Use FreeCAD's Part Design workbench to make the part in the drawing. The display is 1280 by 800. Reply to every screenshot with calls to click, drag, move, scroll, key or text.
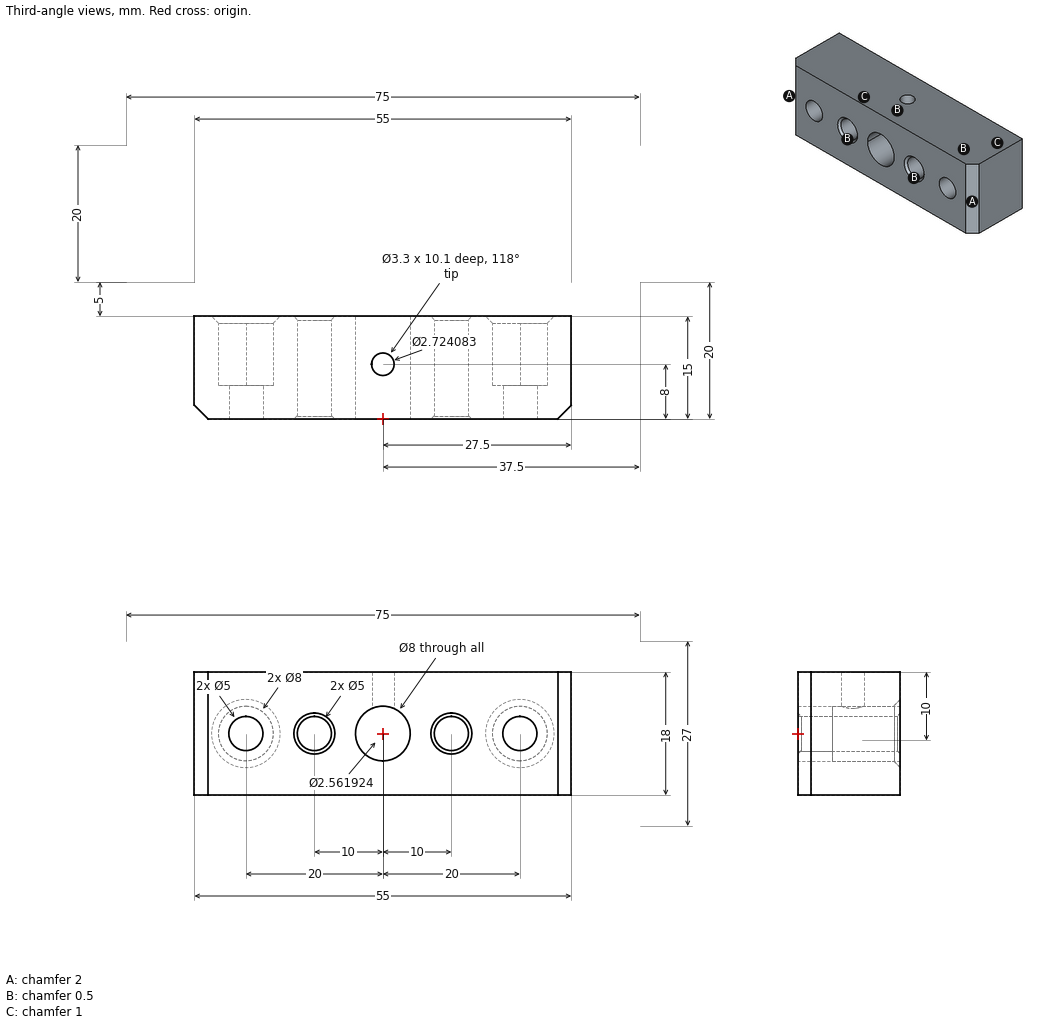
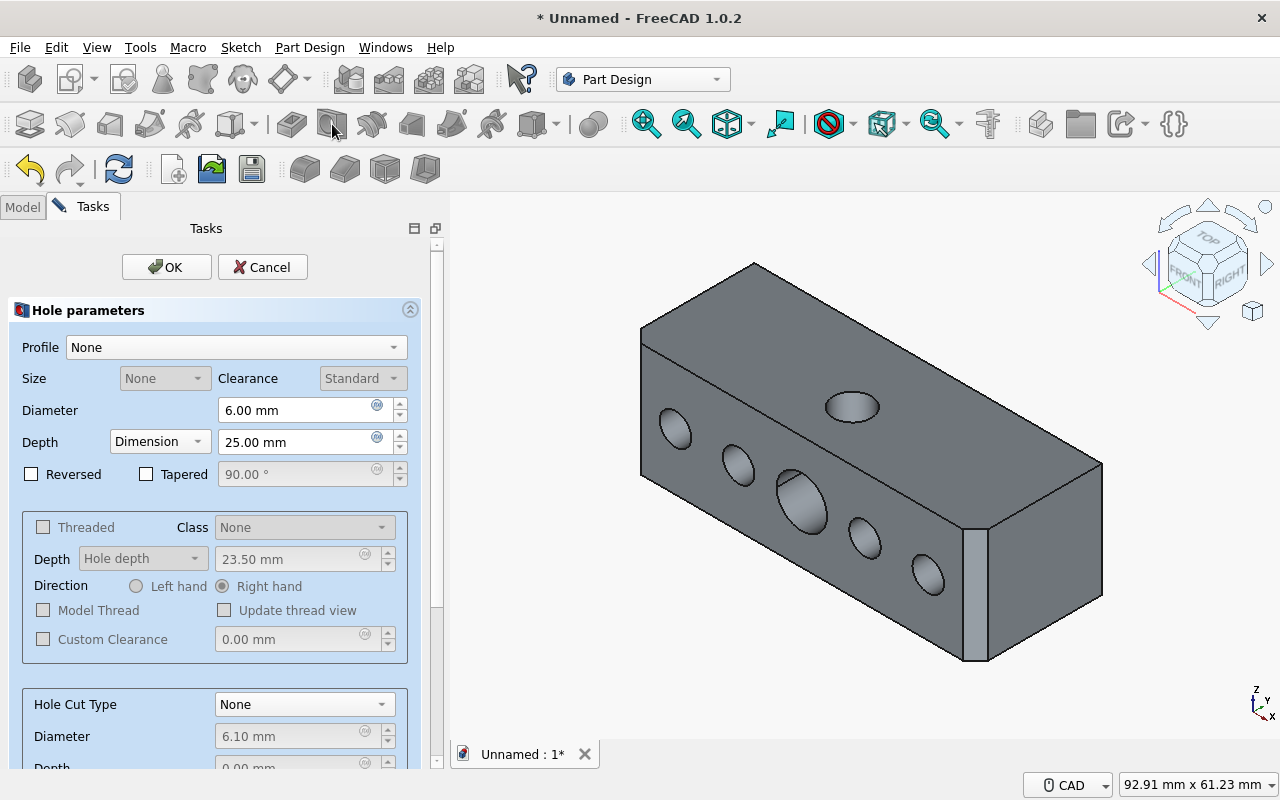
triple_click(305, 410)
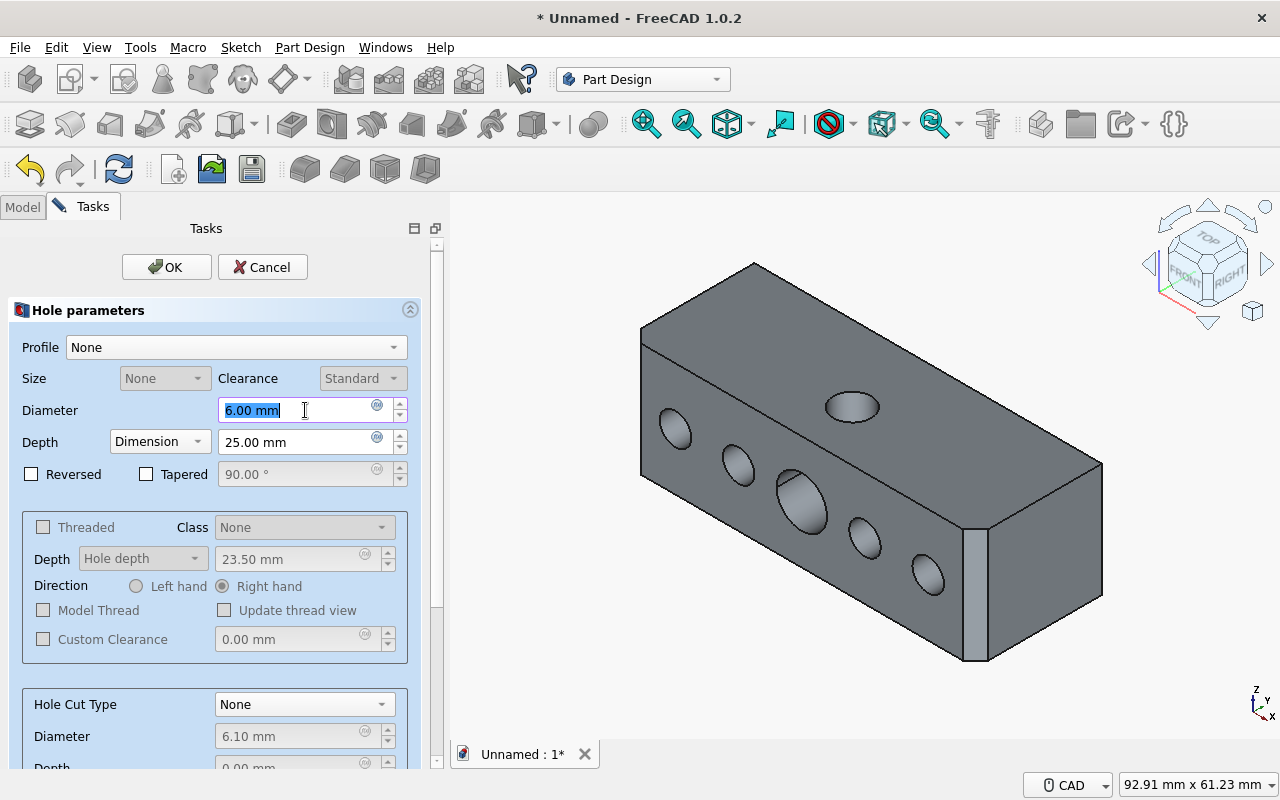
text(3.3)
key(Tab)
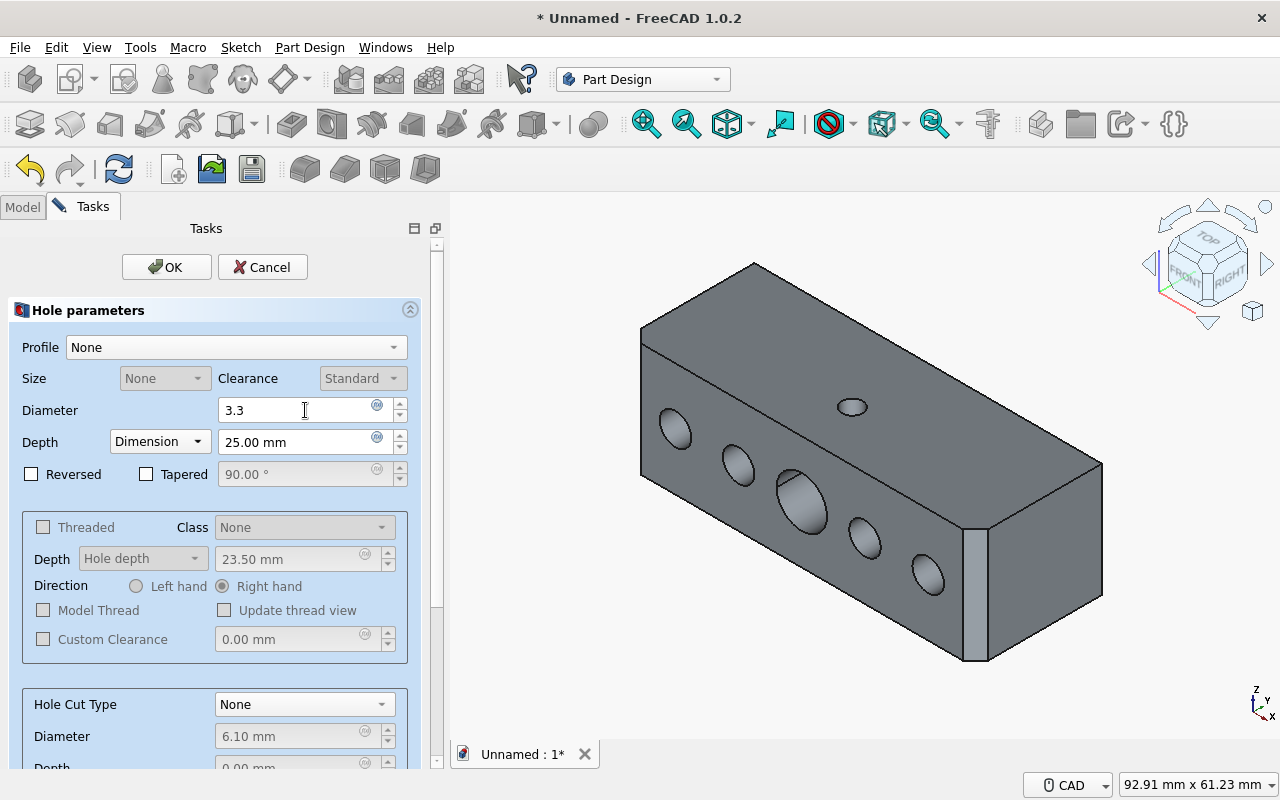
triple_click(305, 442)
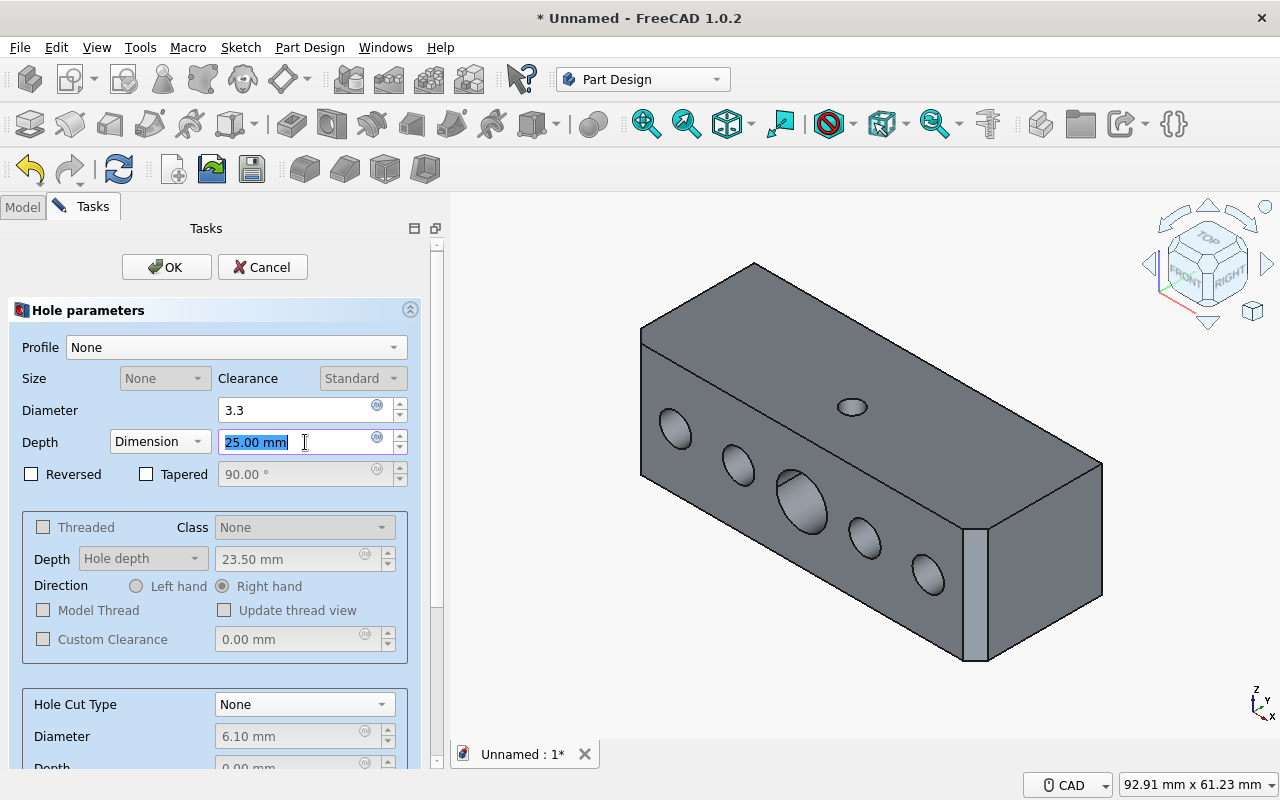
text(10.1)
key(Tab)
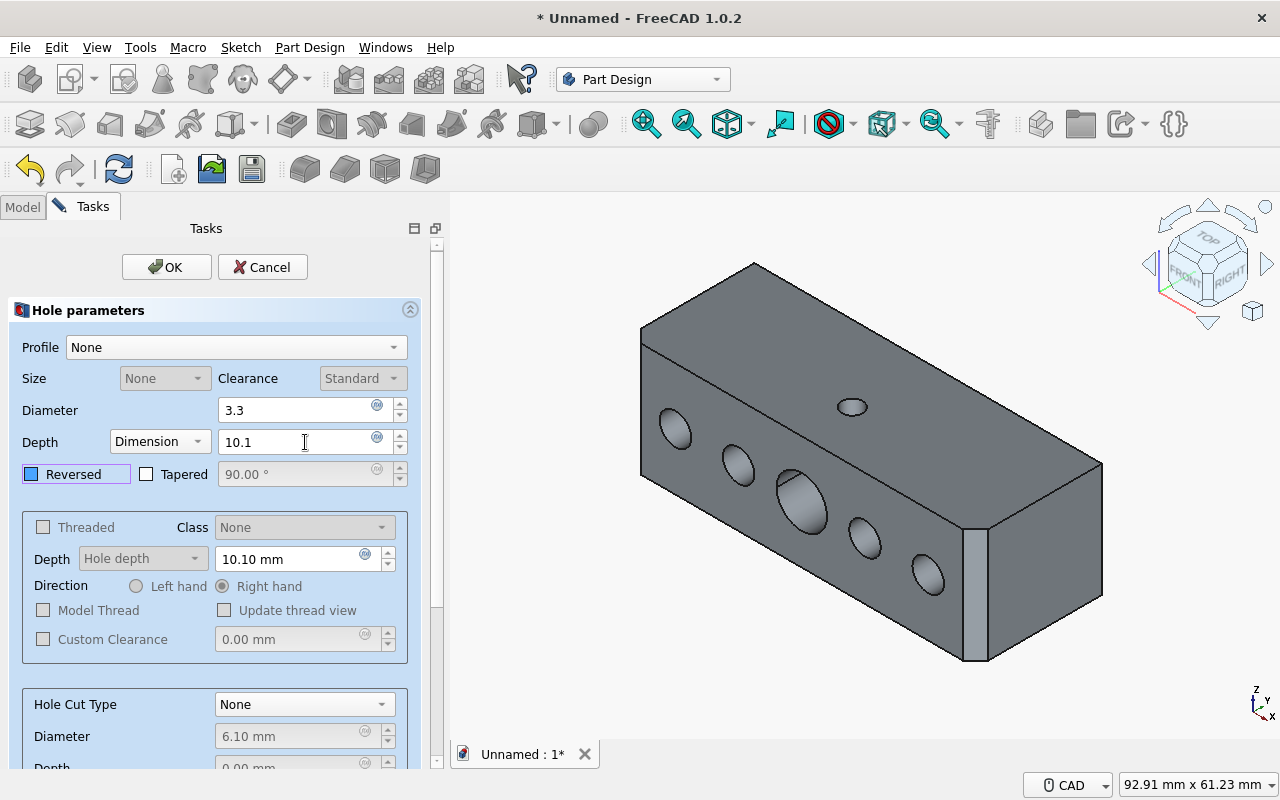
click(167, 267)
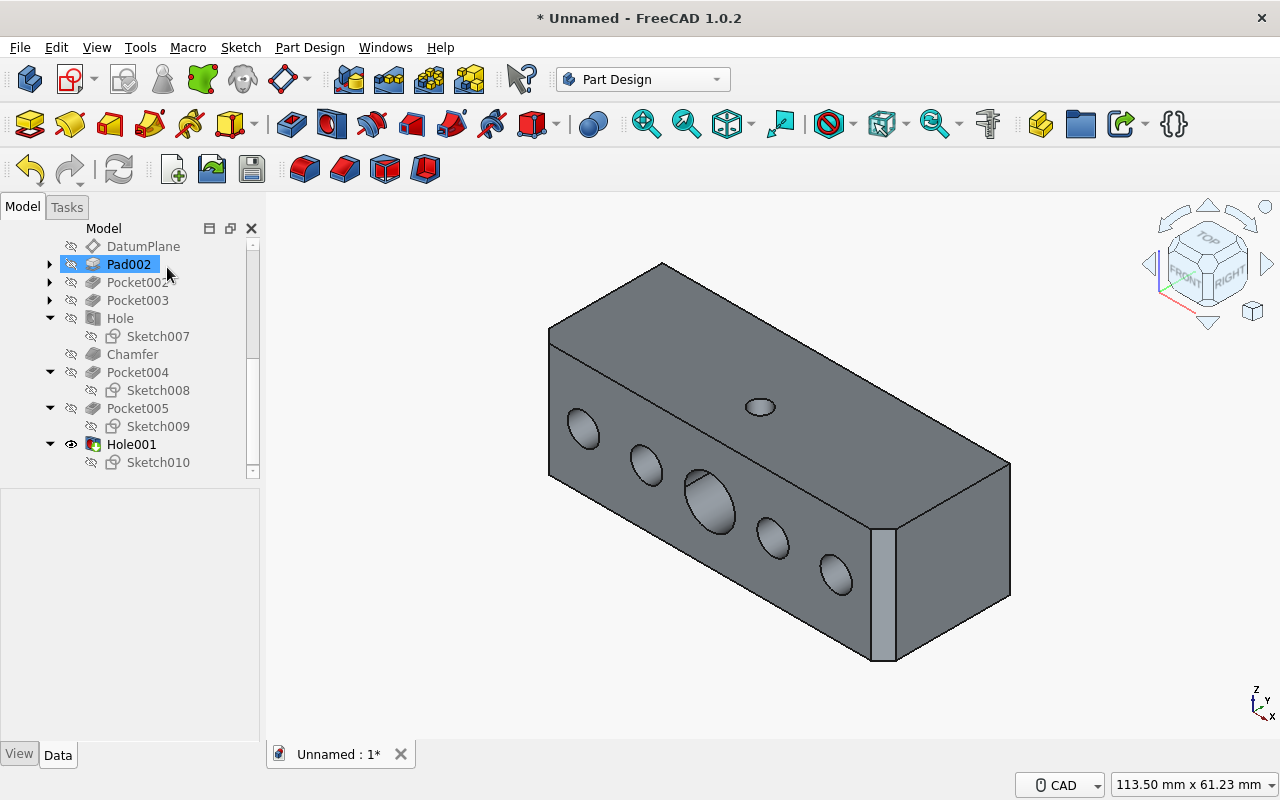
click(872, 456)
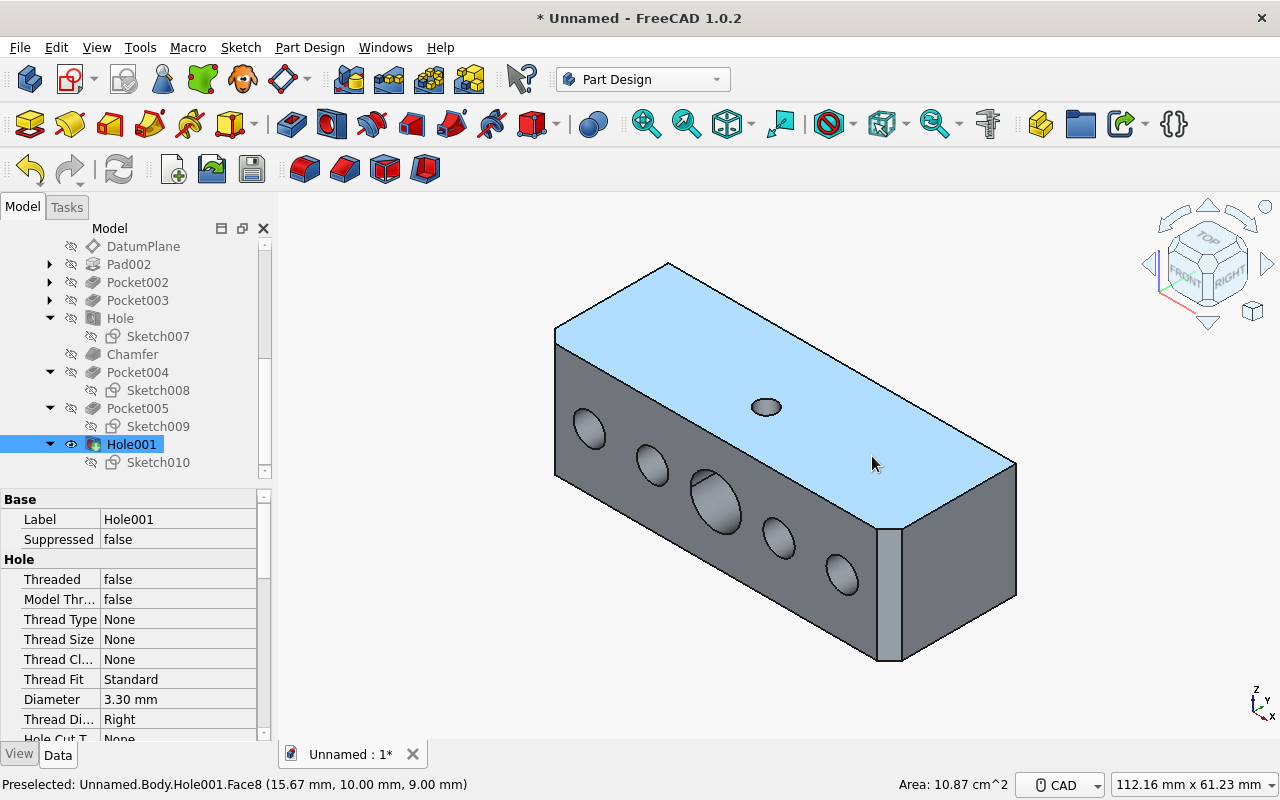
click(70, 80)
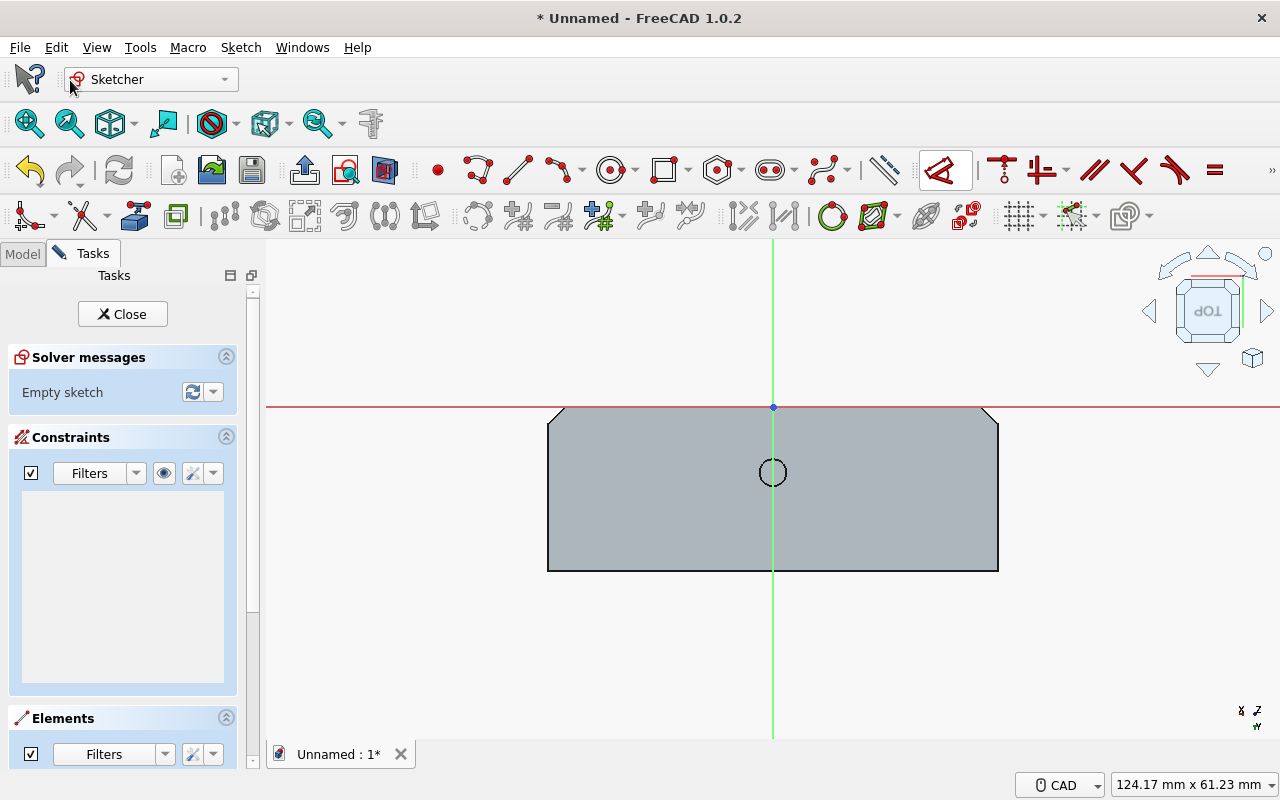
click(664, 170)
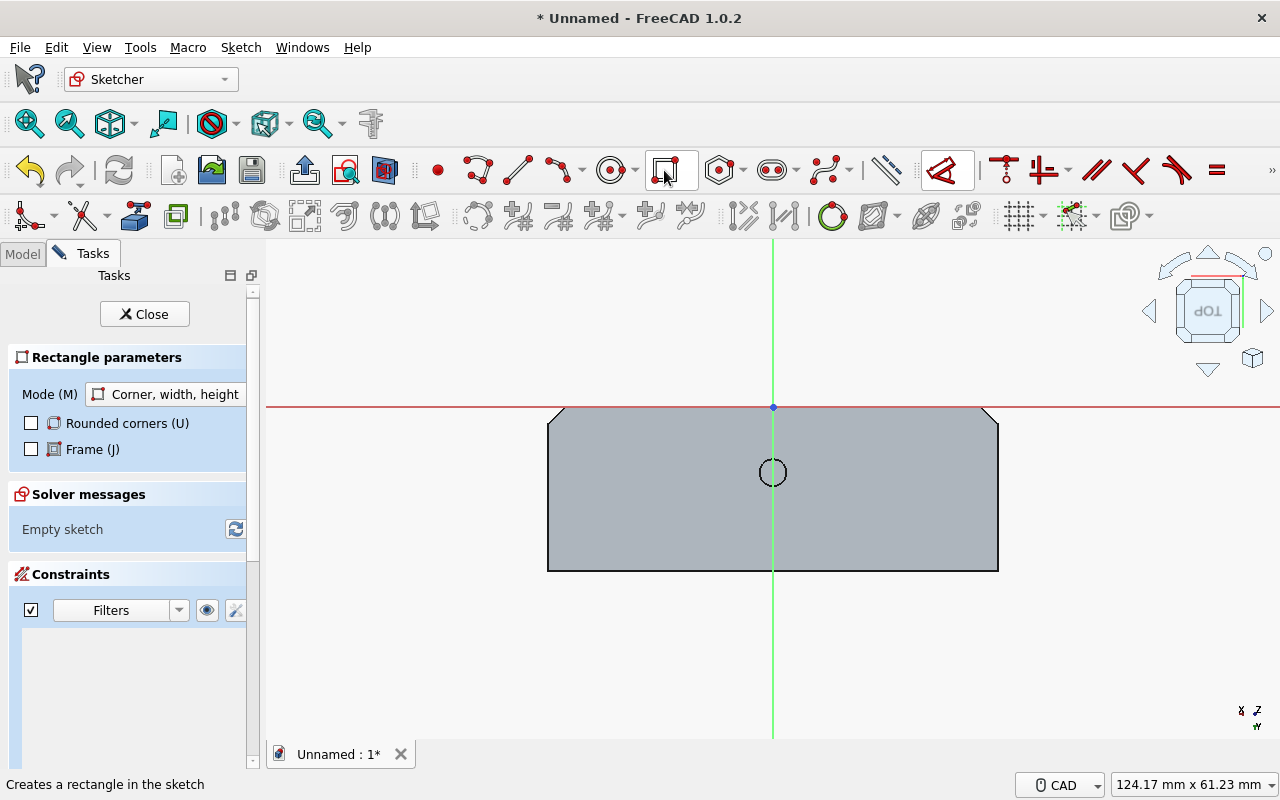
click(548, 530)
move(998, 571)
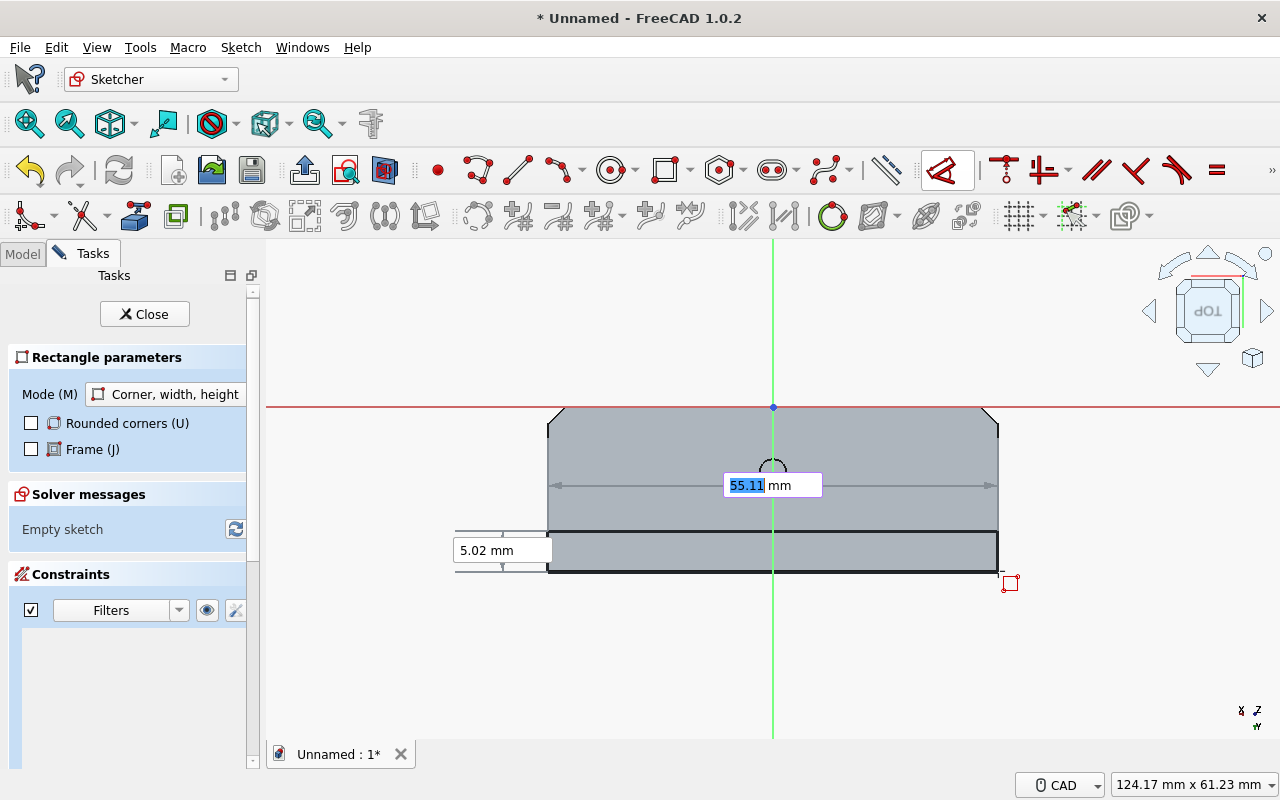
text(55)
key(Tab)
text(5)
key(Return)
key(Escape)